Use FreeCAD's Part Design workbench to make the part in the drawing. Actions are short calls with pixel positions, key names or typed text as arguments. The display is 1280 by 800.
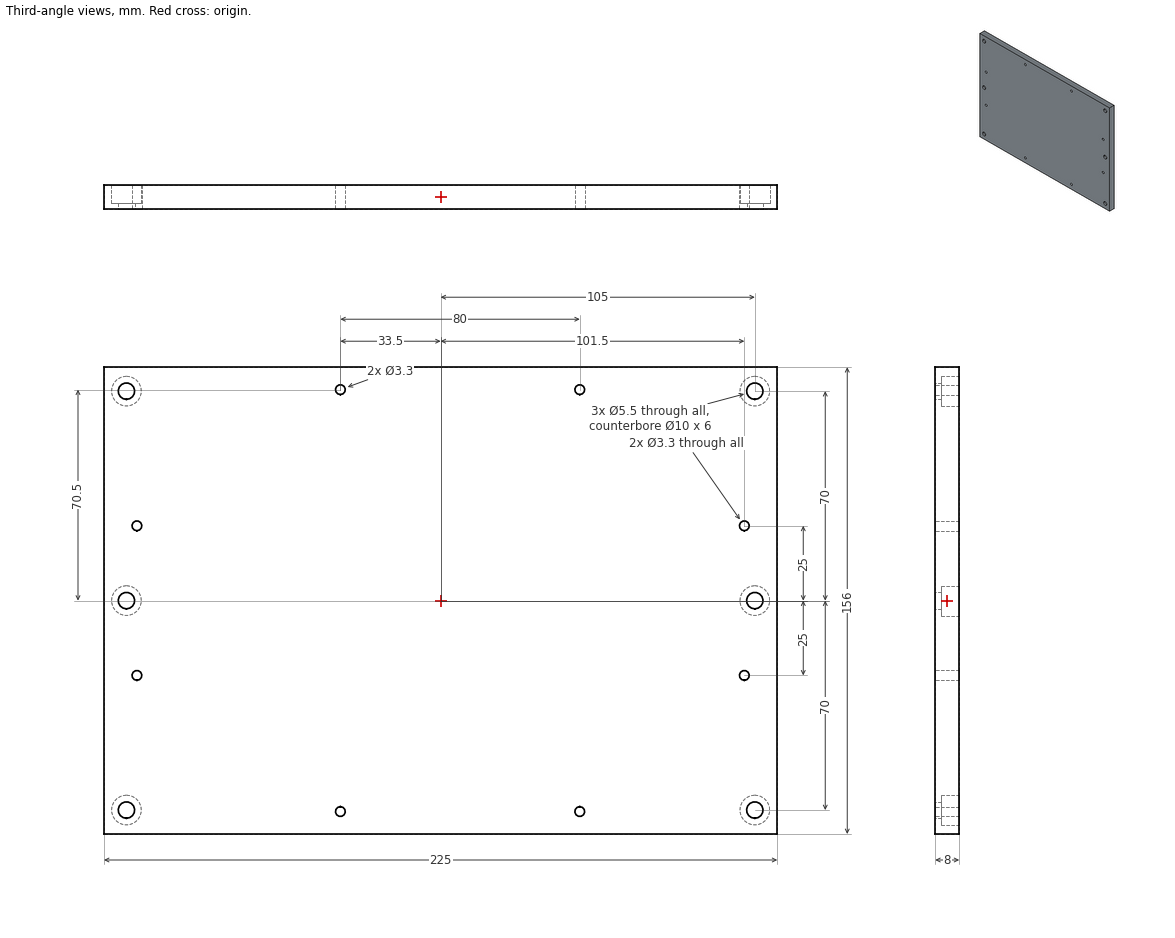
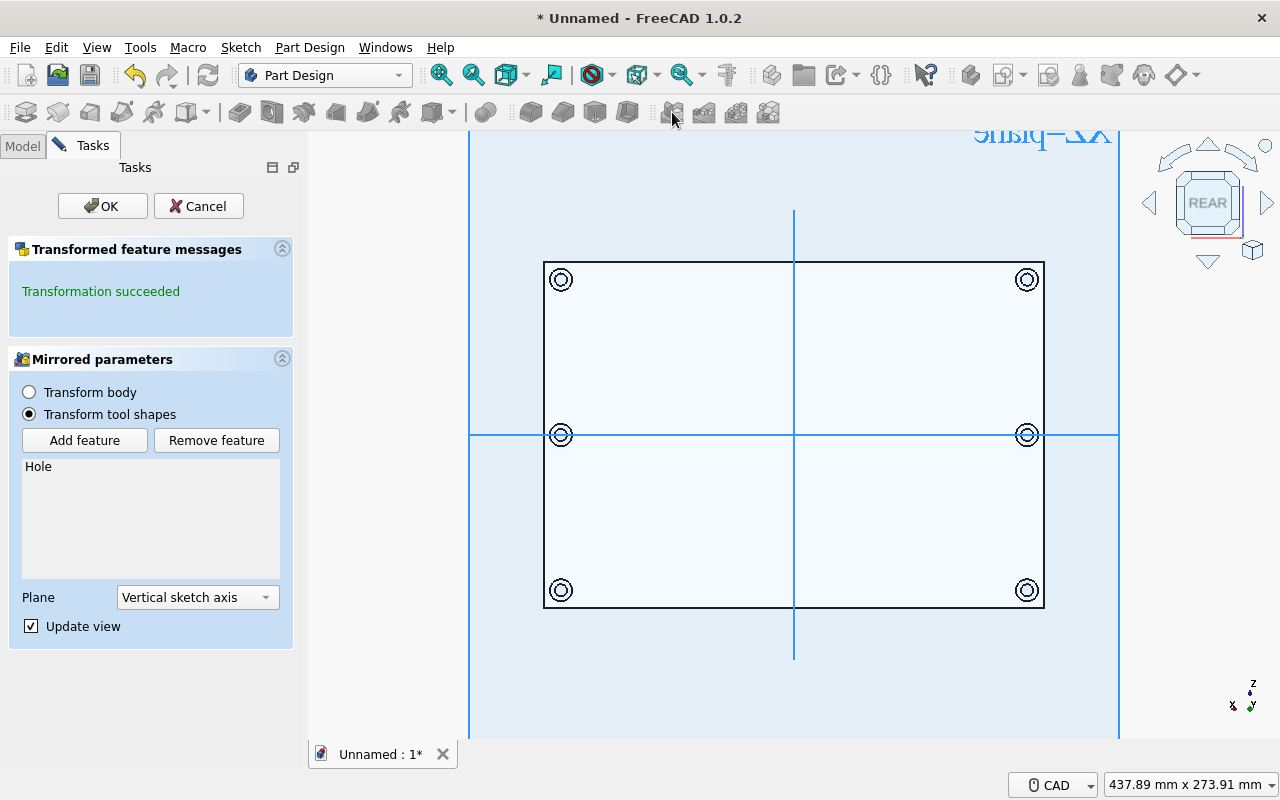
click(198, 598)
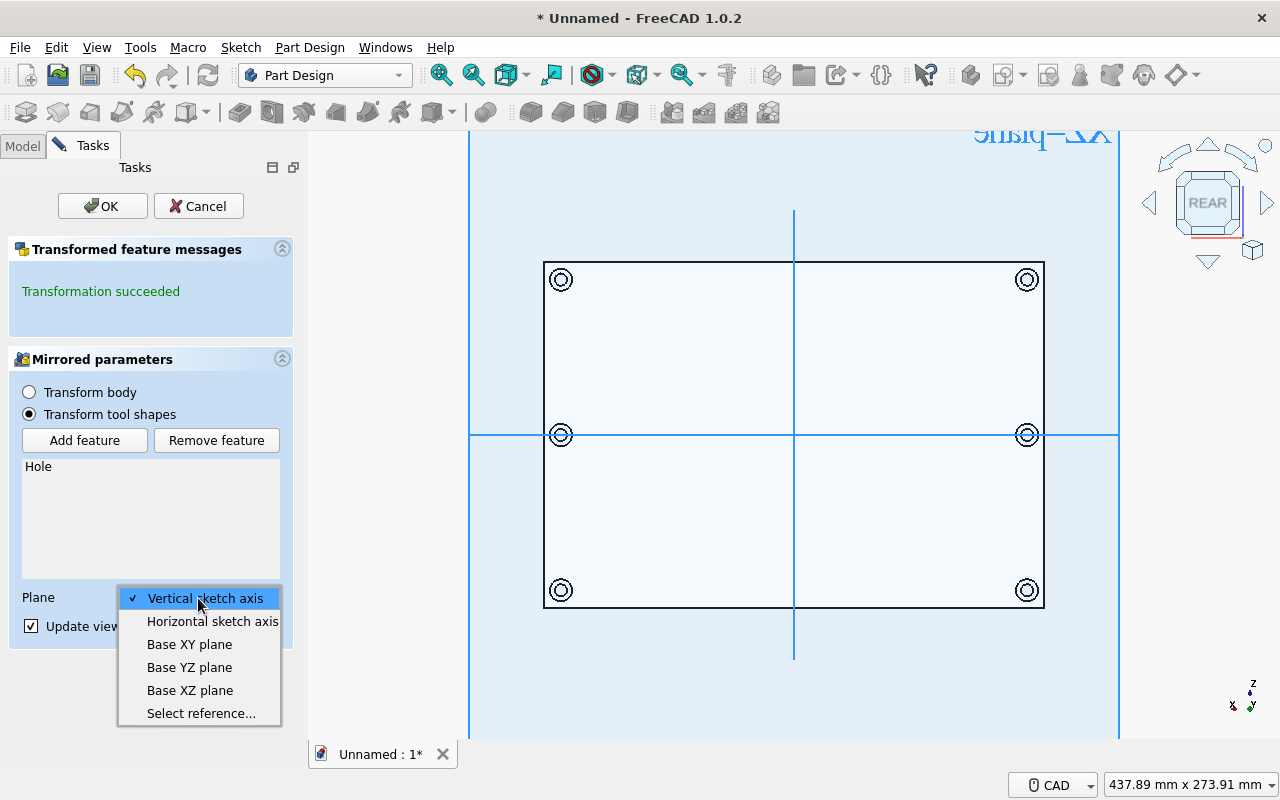
click(198, 668)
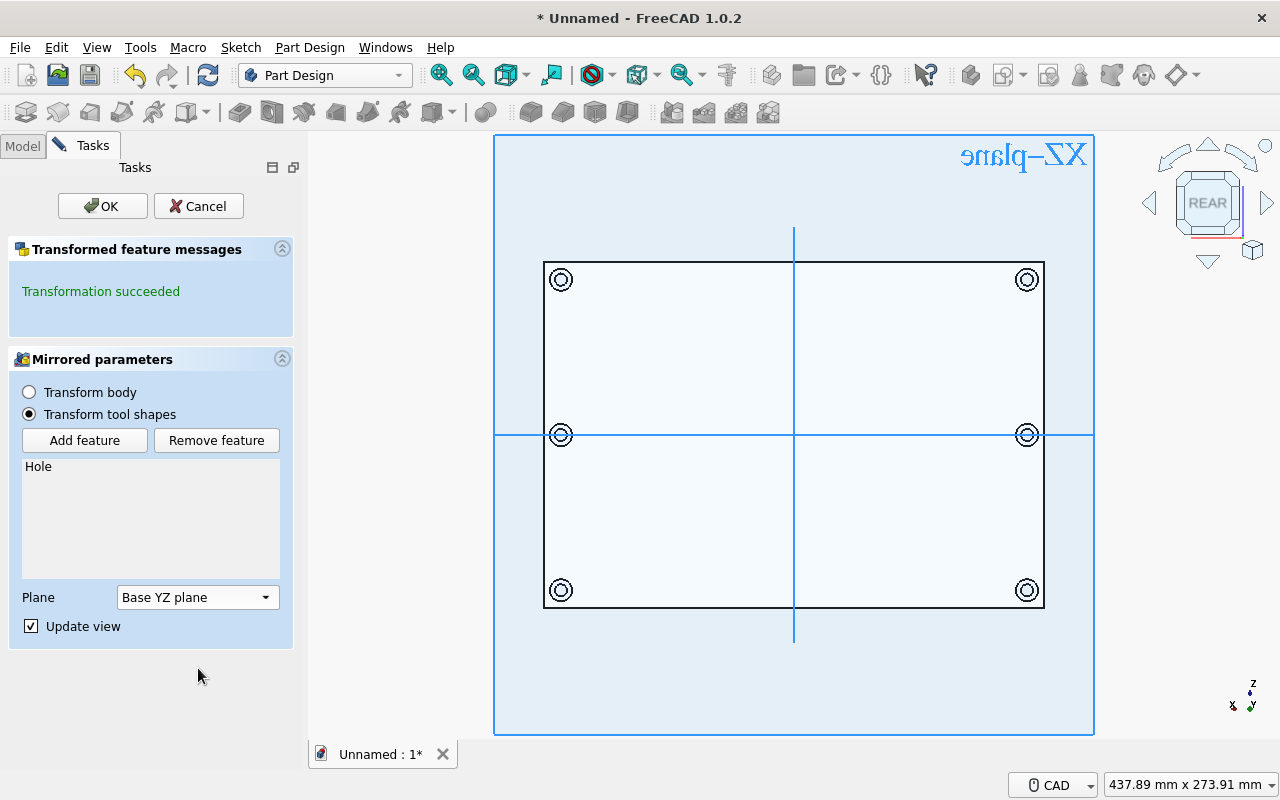
click(103, 206)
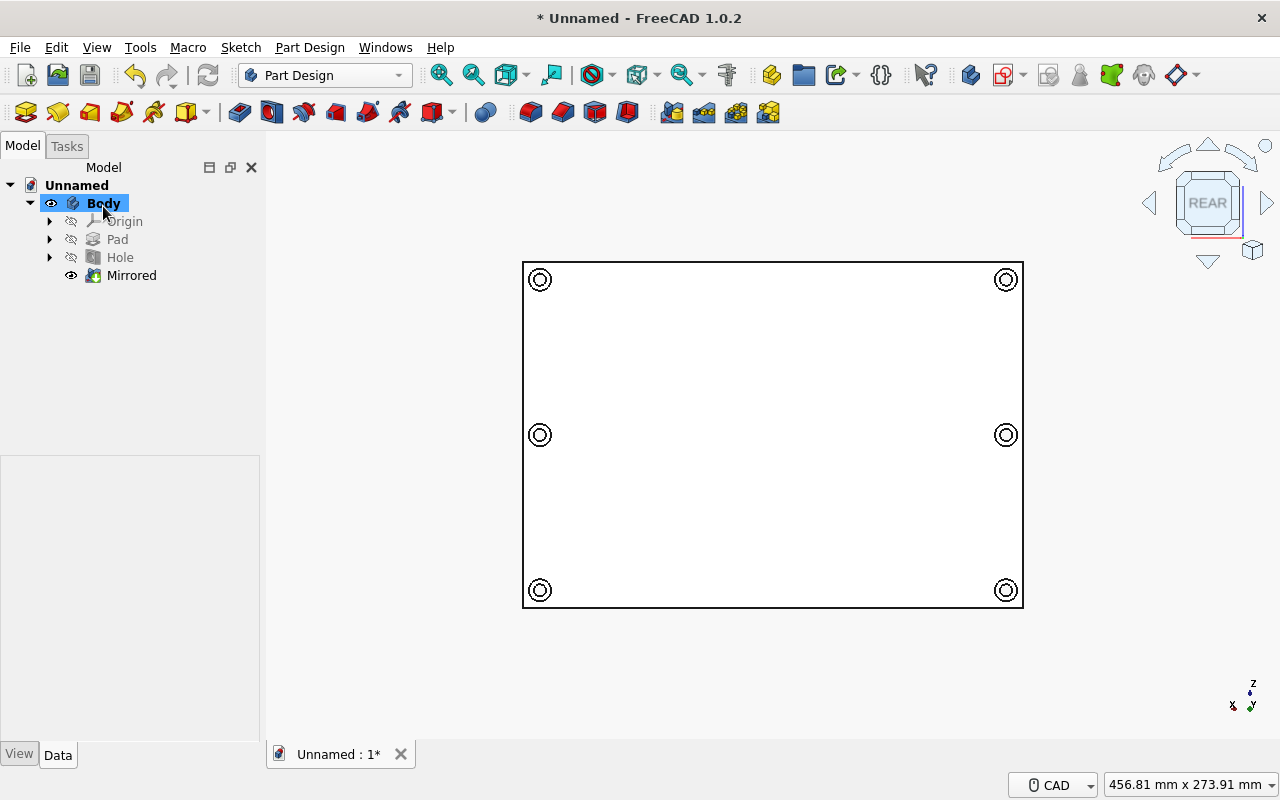
click(773, 434)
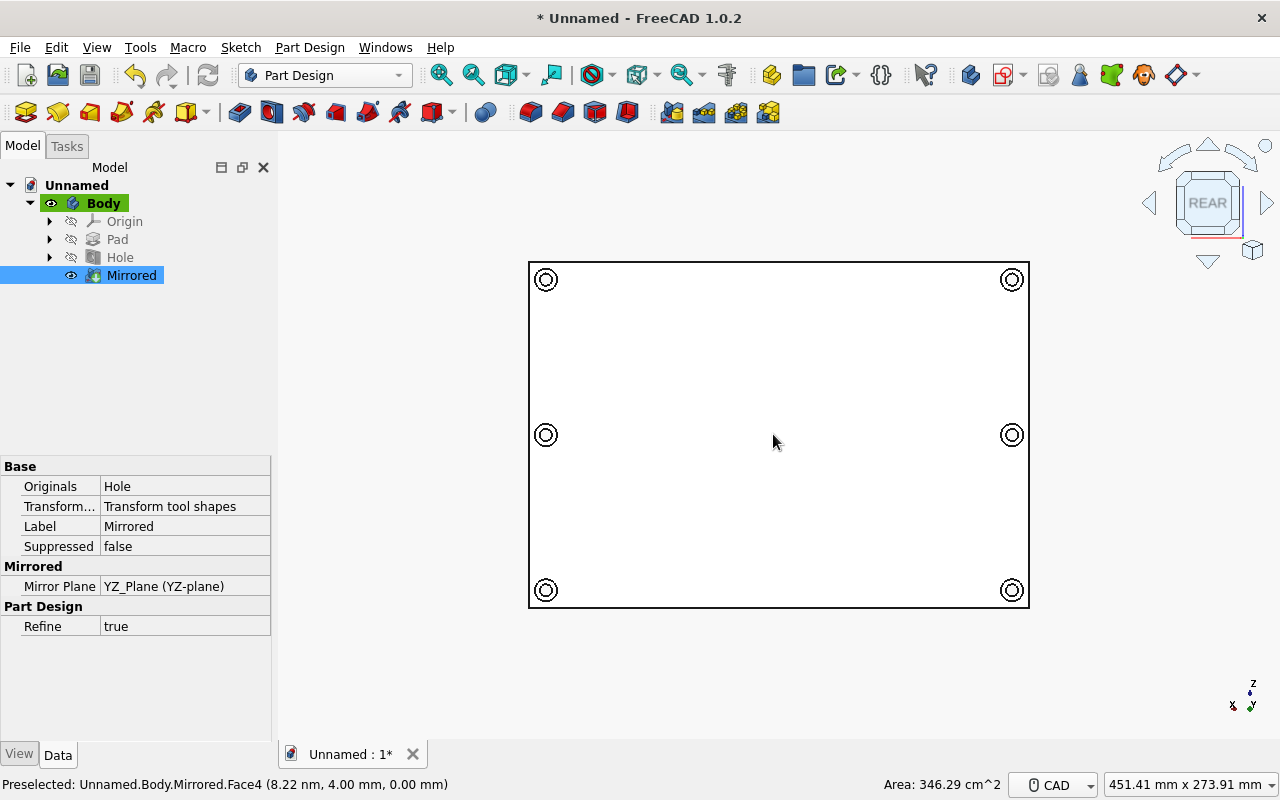
click(1004, 76)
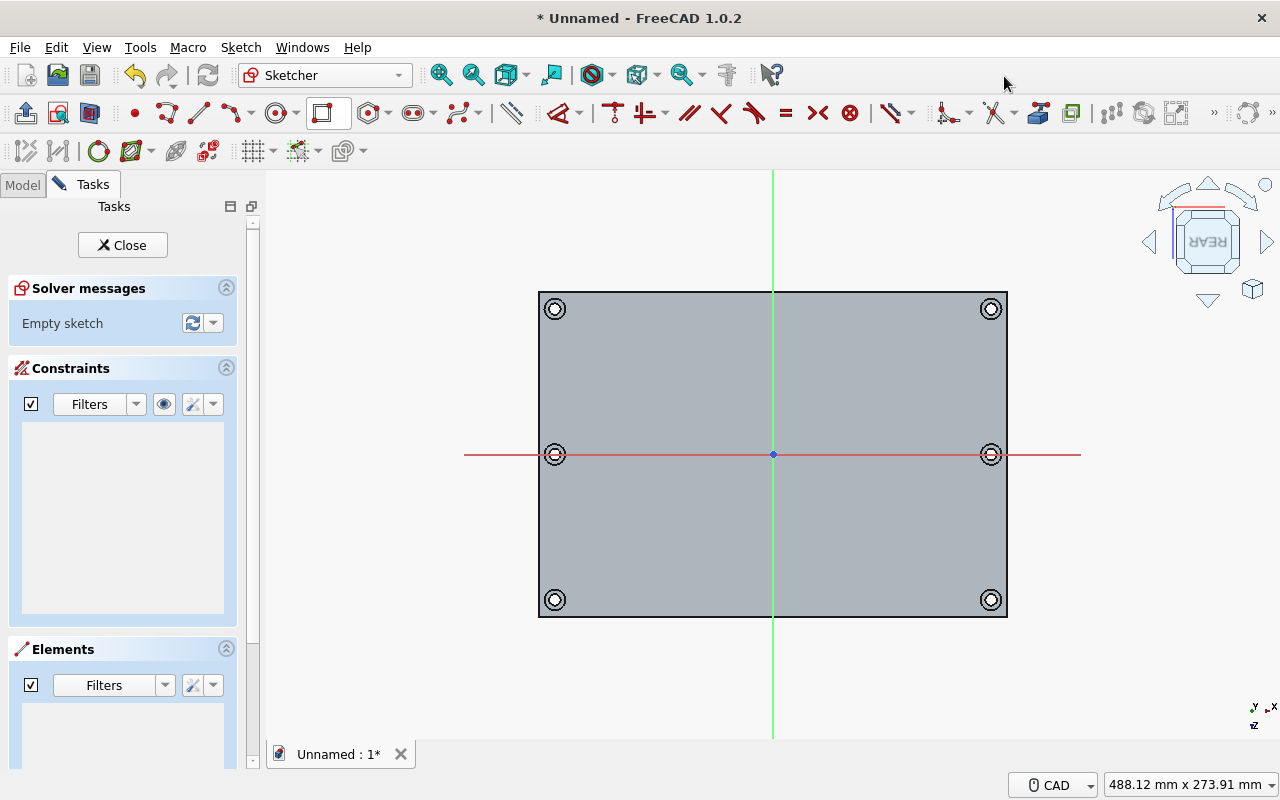
scroll(982, 454, up, 5)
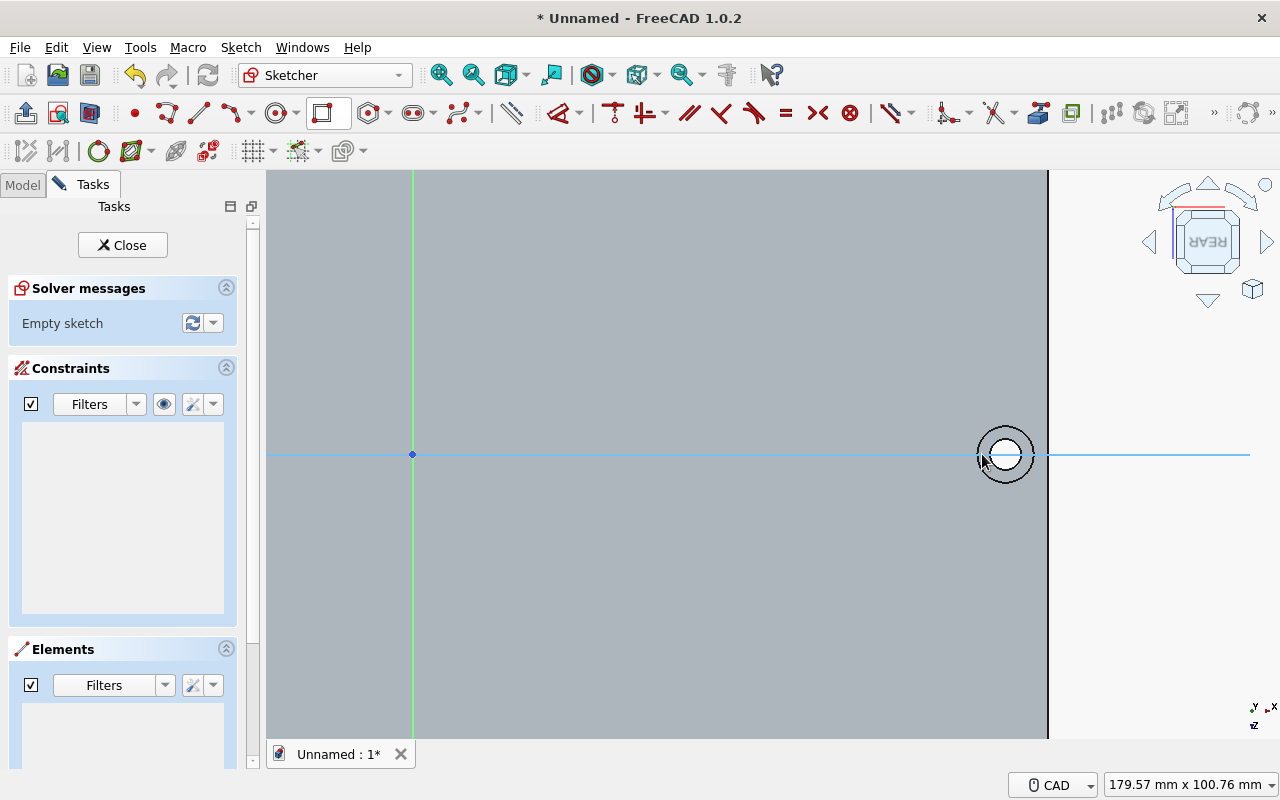
key(g)
key(c)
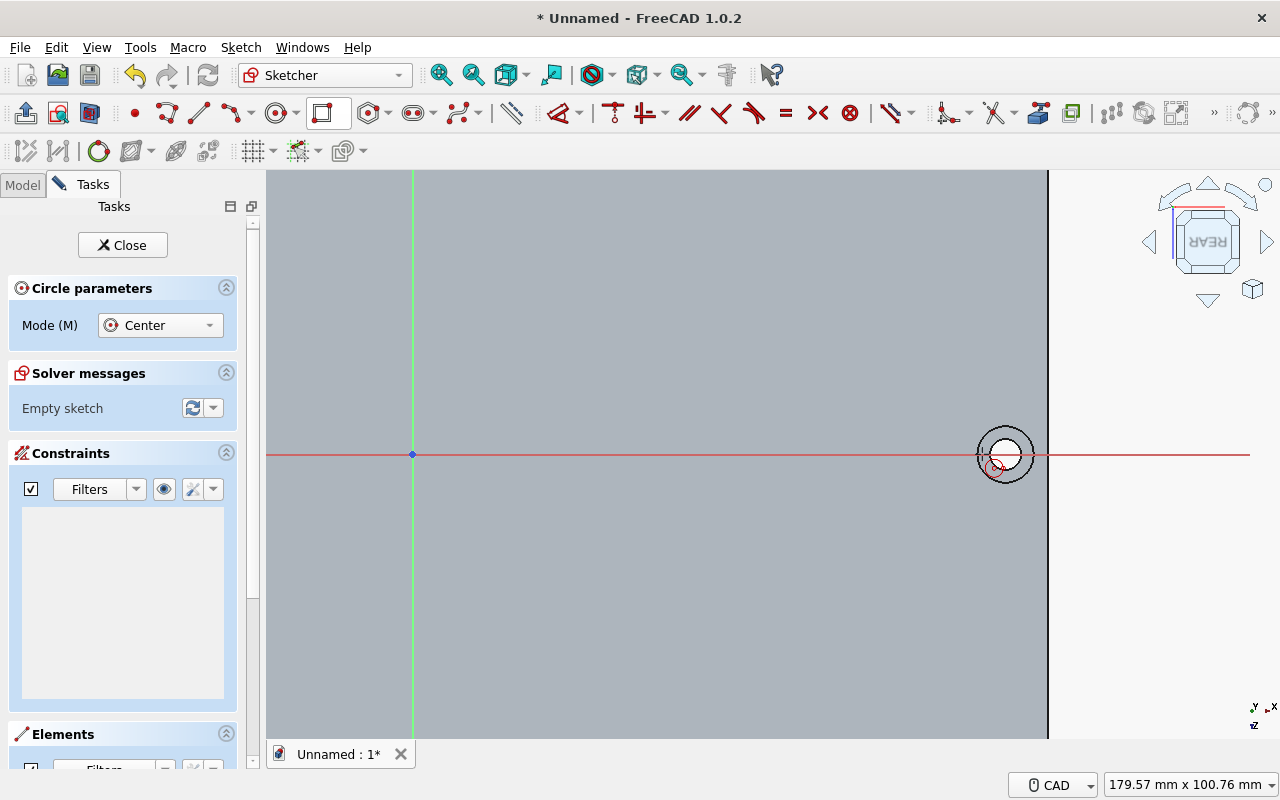
scroll(986, 596, up, 5)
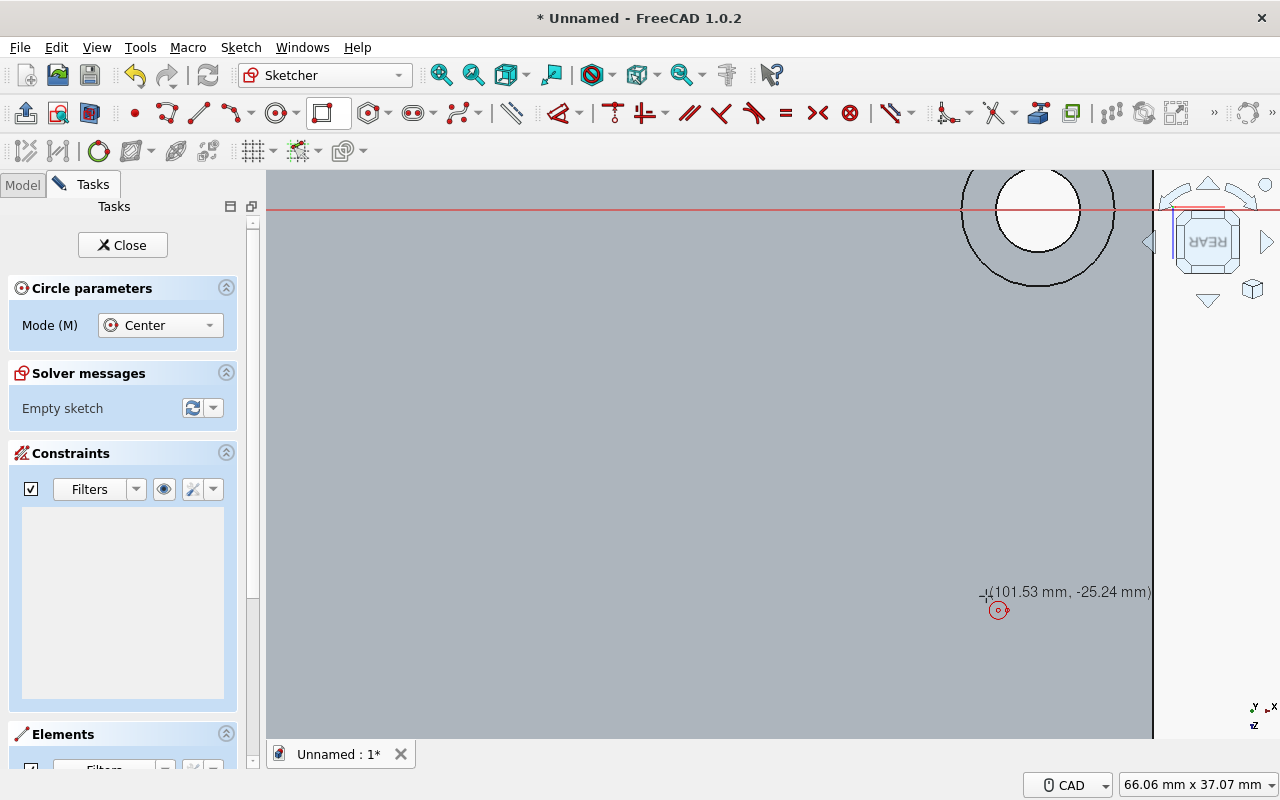
click(984, 594)
click(1002, 576)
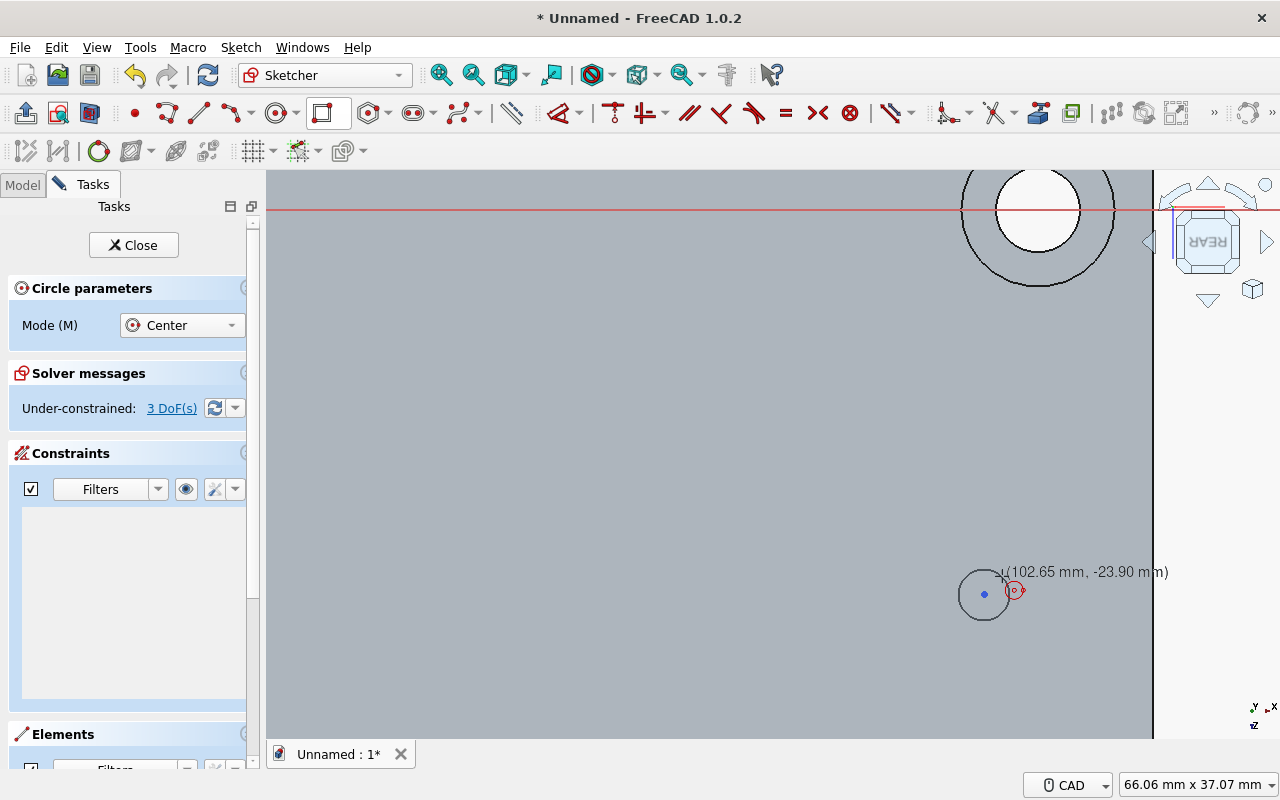
scroll(988, 597, down, 5)